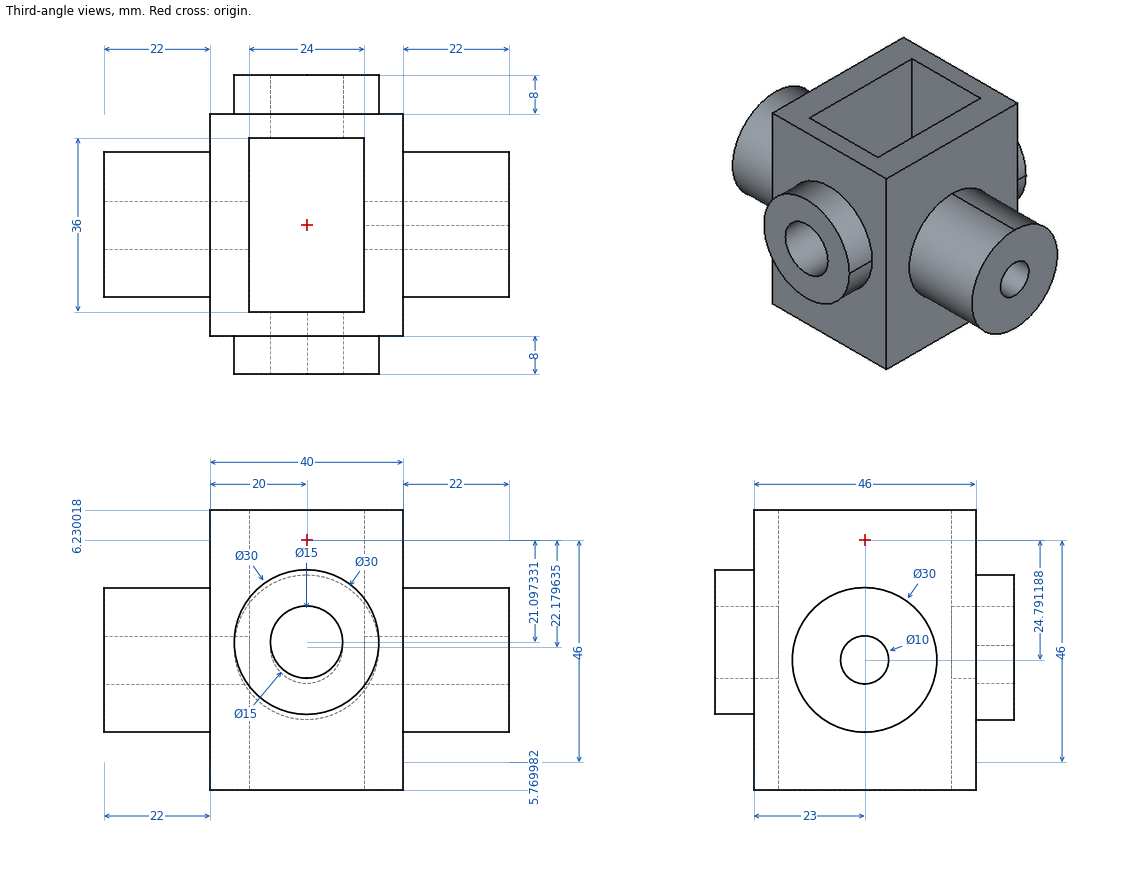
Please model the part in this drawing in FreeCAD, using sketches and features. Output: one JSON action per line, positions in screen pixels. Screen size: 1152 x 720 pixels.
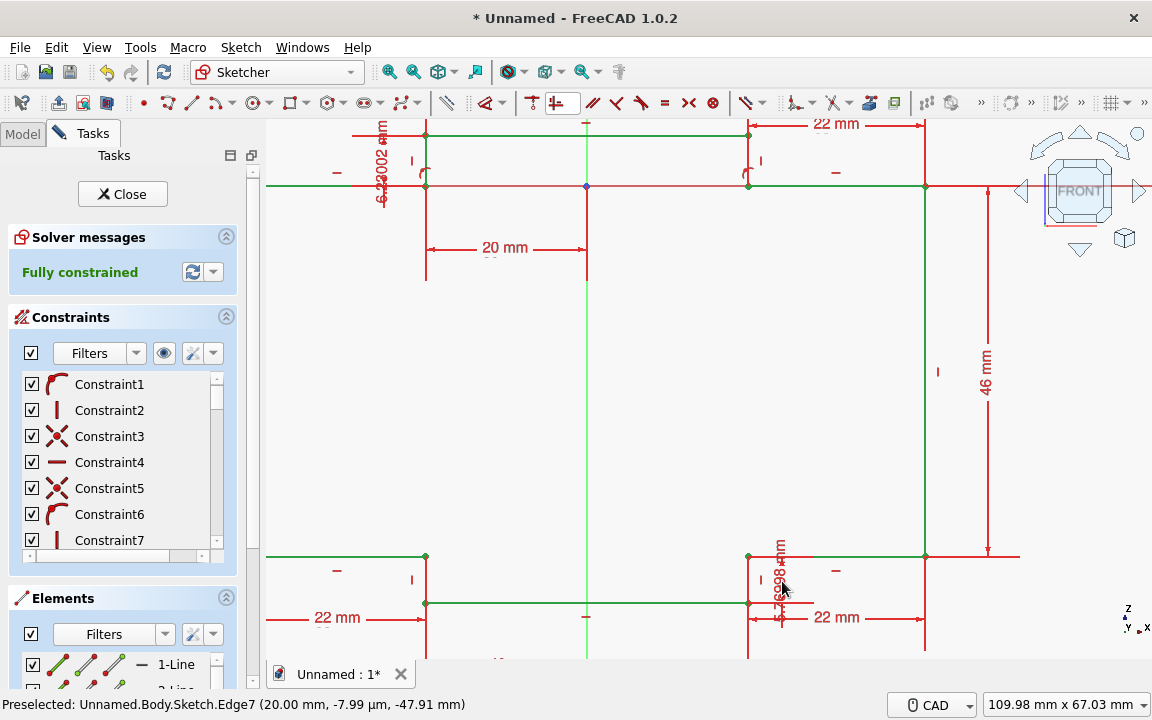
{"action": "left_click", "coordinate": [123, 194]}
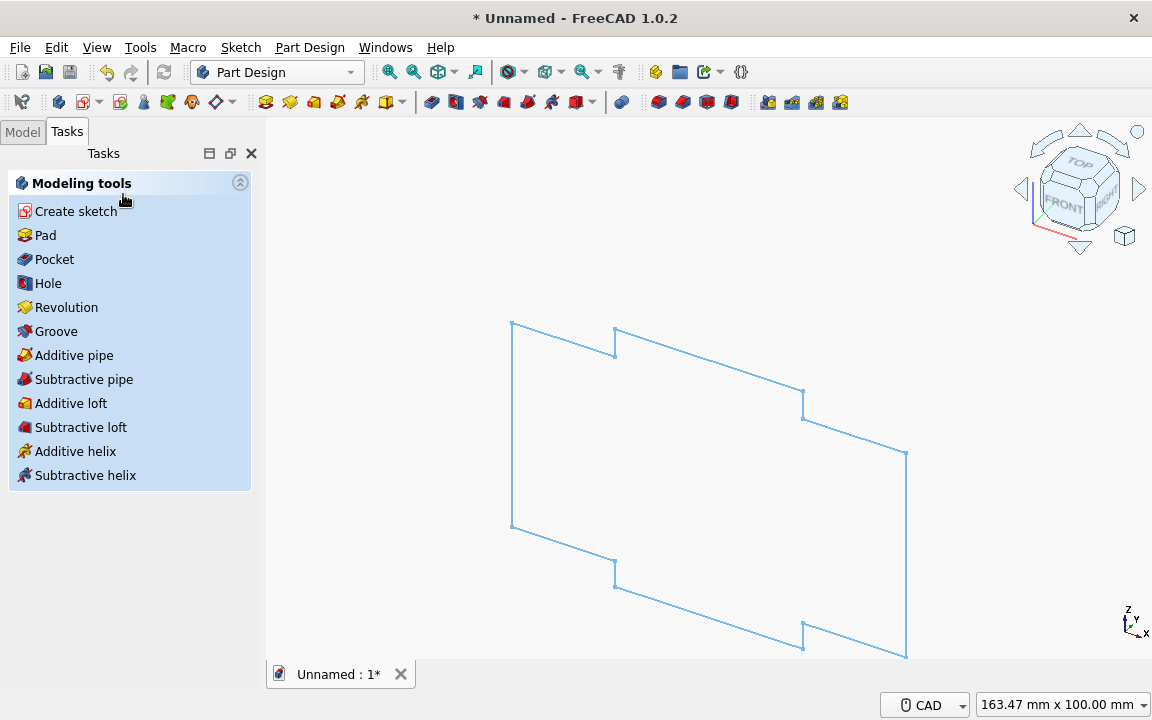
{"action": "left_click", "coordinate": [266, 102]}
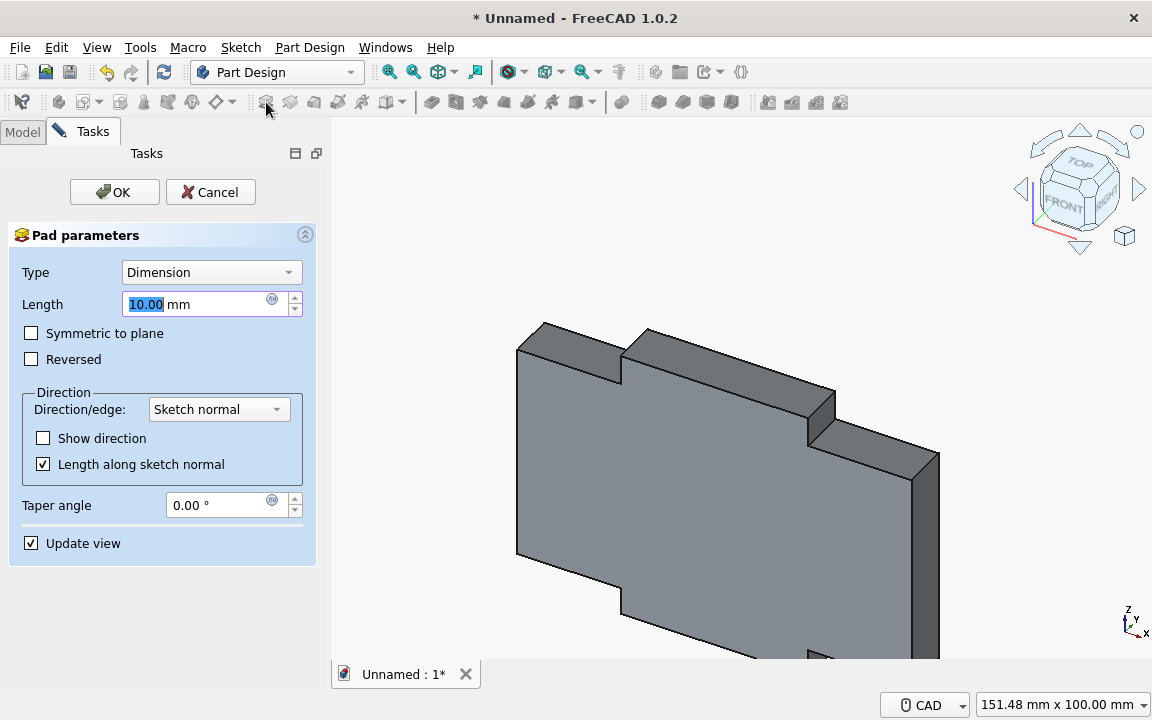
{"action": "type", "text": "46"}
{"action": "key", "text": "Tab"}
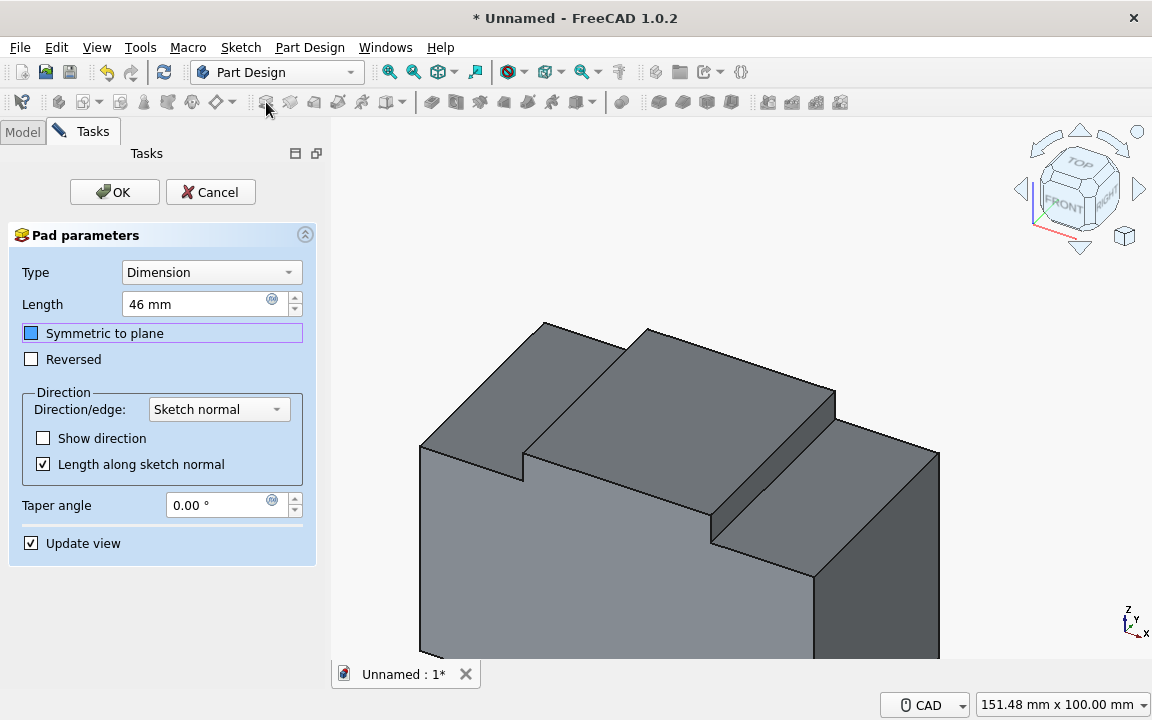
{"action": "left_click", "coordinate": [30, 333]}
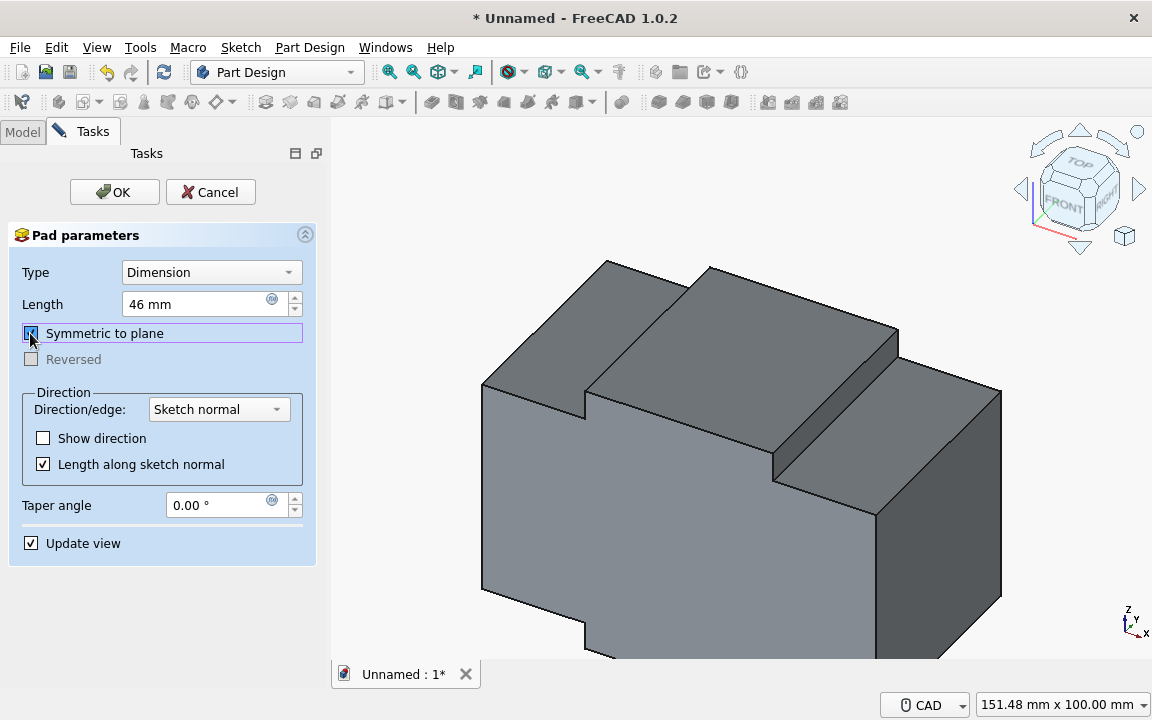
{"action": "left_click", "coordinate": [115, 192]}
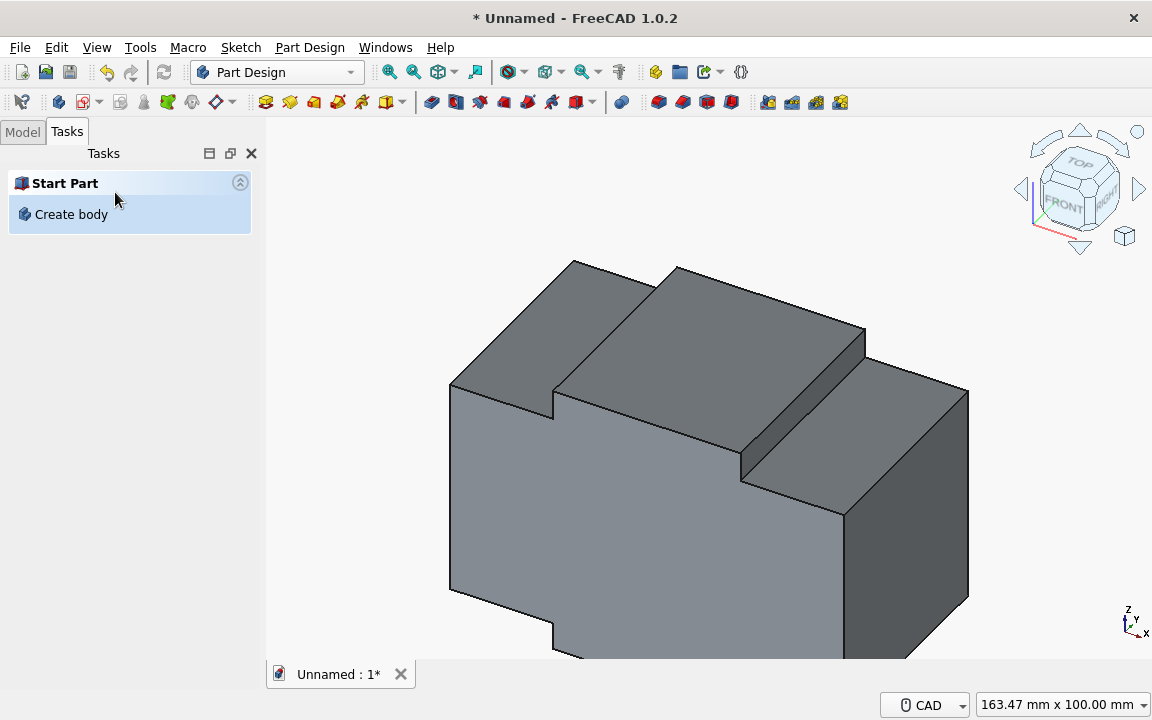
{"action": "left_click", "coordinate": [390, 72]}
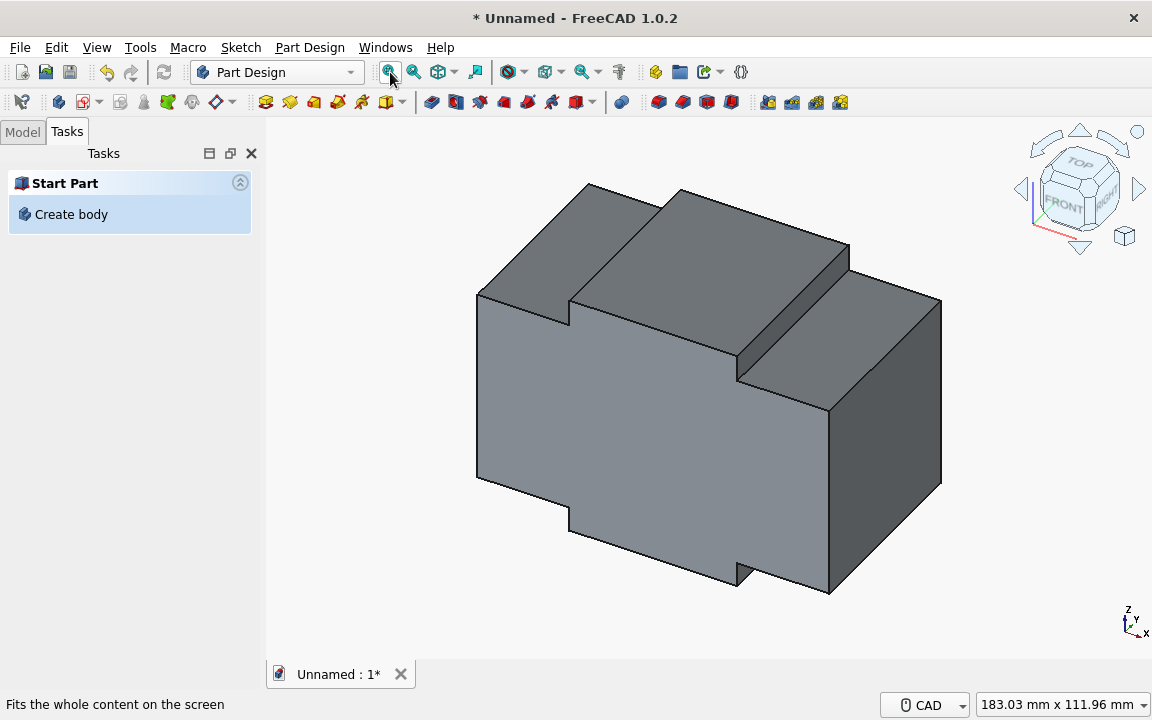
{"action": "key", "text": "4"}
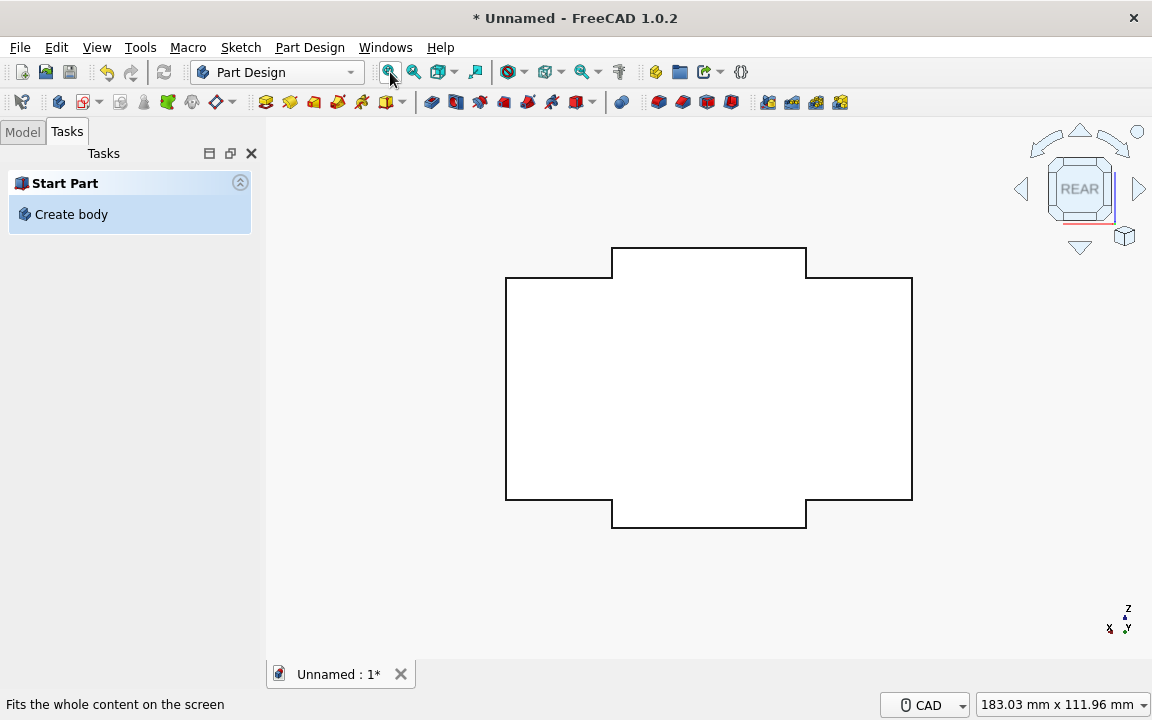
{"action": "left_click", "coordinate": [709, 387]}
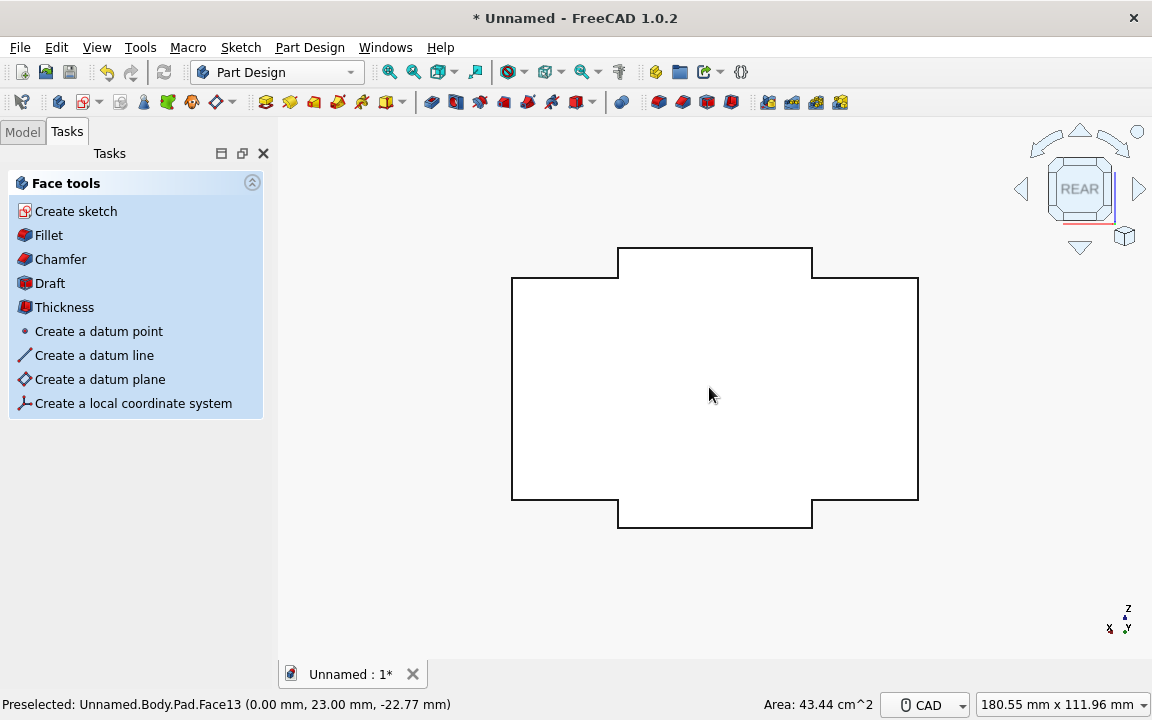
{"action": "left_click", "coordinate": [84, 102]}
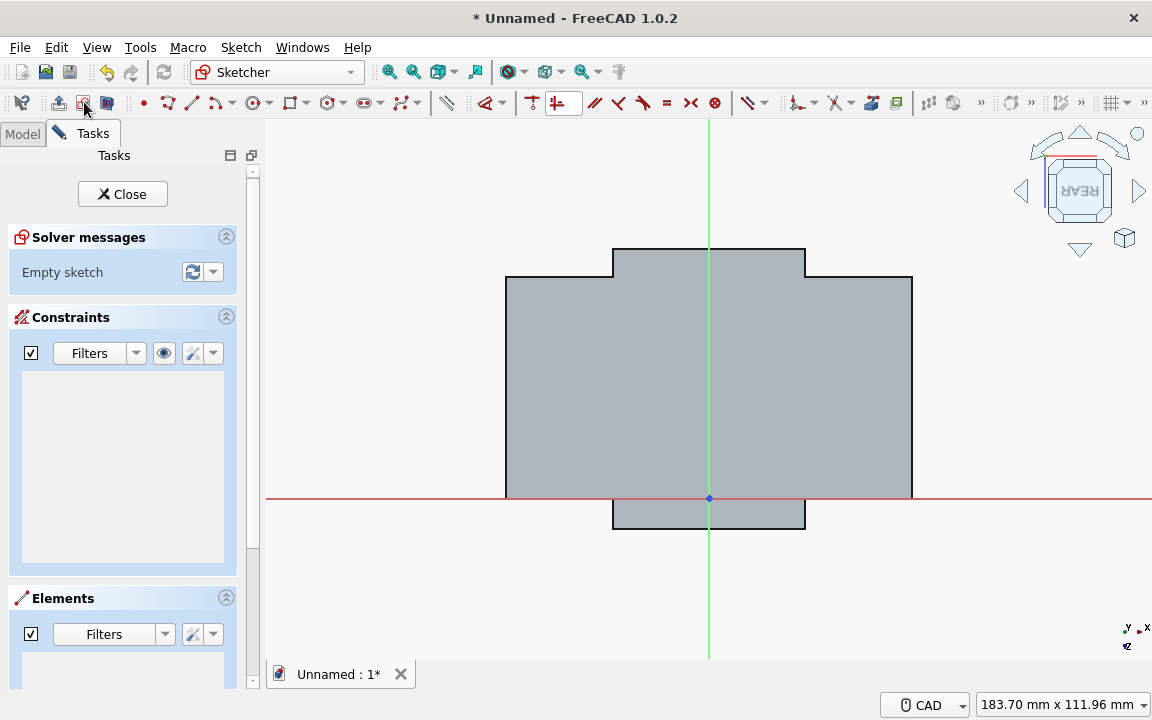
{"action": "scroll", "coordinate": [792, 434], "scroll_direction": "up", "scroll_amount": 3}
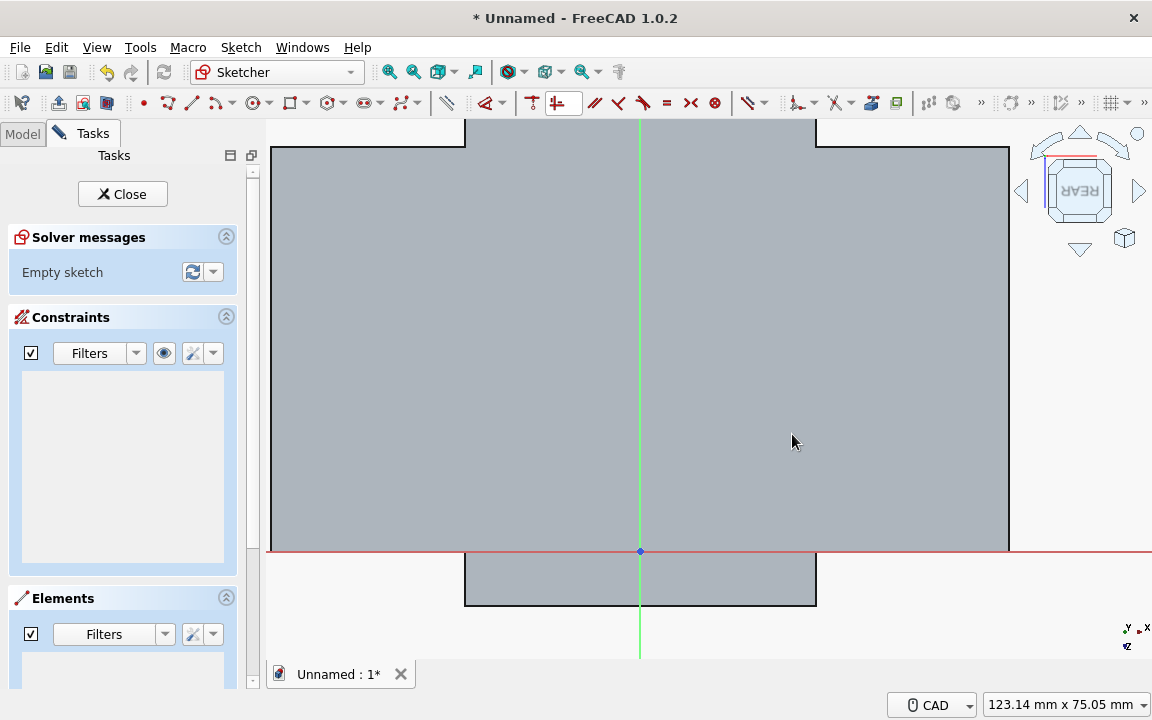
{"action": "left_click", "coordinate": [254, 104]}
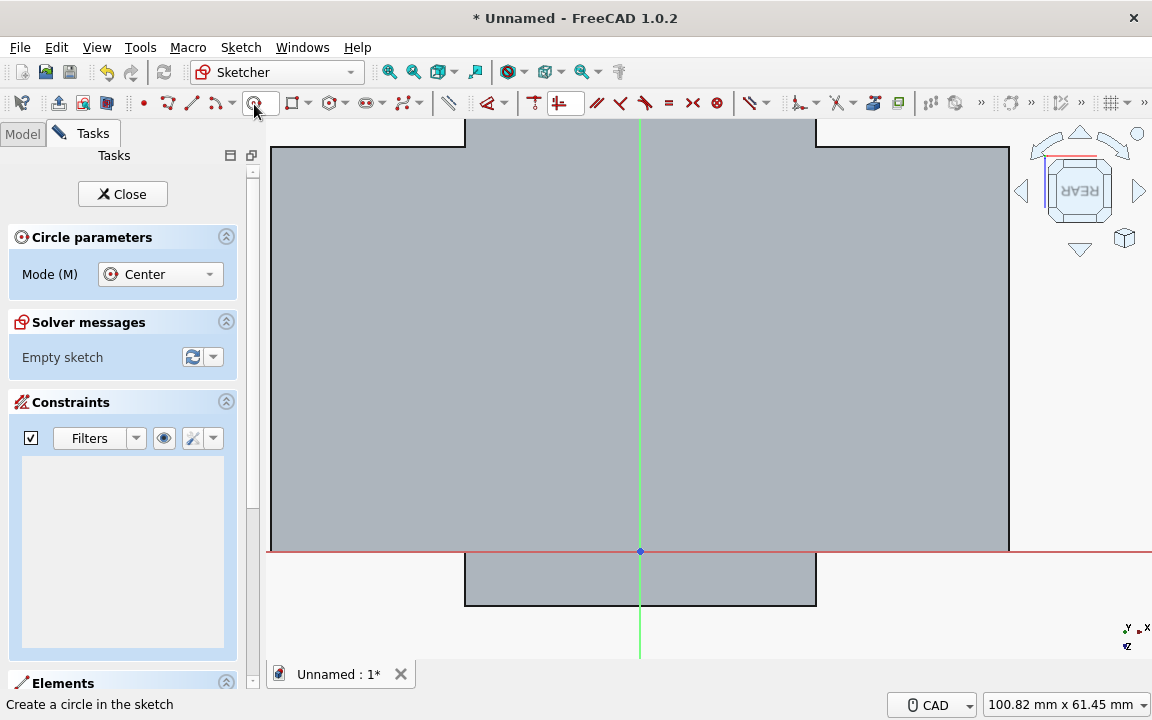
{"action": "left_click", "coordinate": [640, 357]}
{"action": "left_click", "coordinate": [733, 264]}